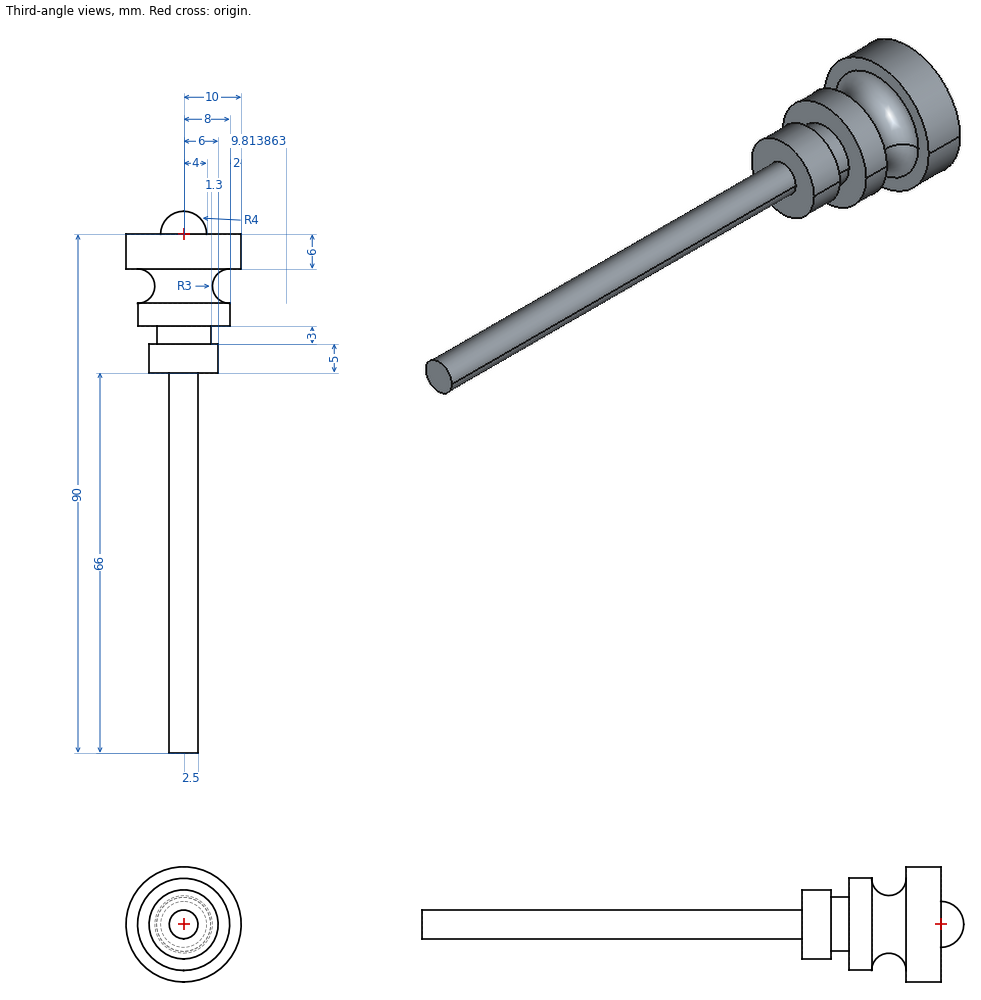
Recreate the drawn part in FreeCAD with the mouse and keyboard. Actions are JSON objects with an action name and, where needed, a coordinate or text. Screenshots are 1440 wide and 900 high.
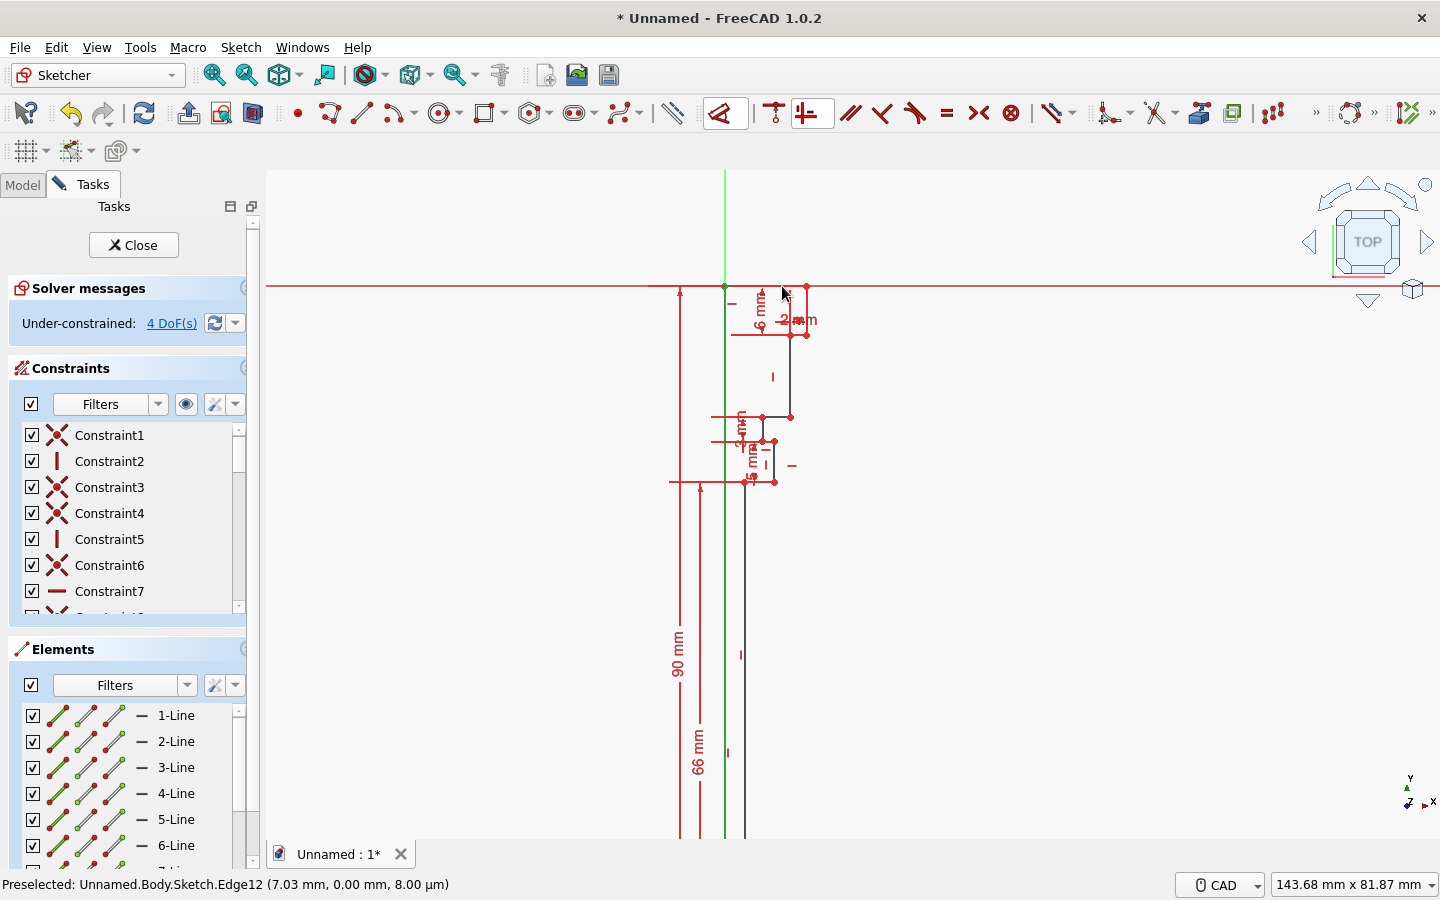
{"action": "key", "text": "l"}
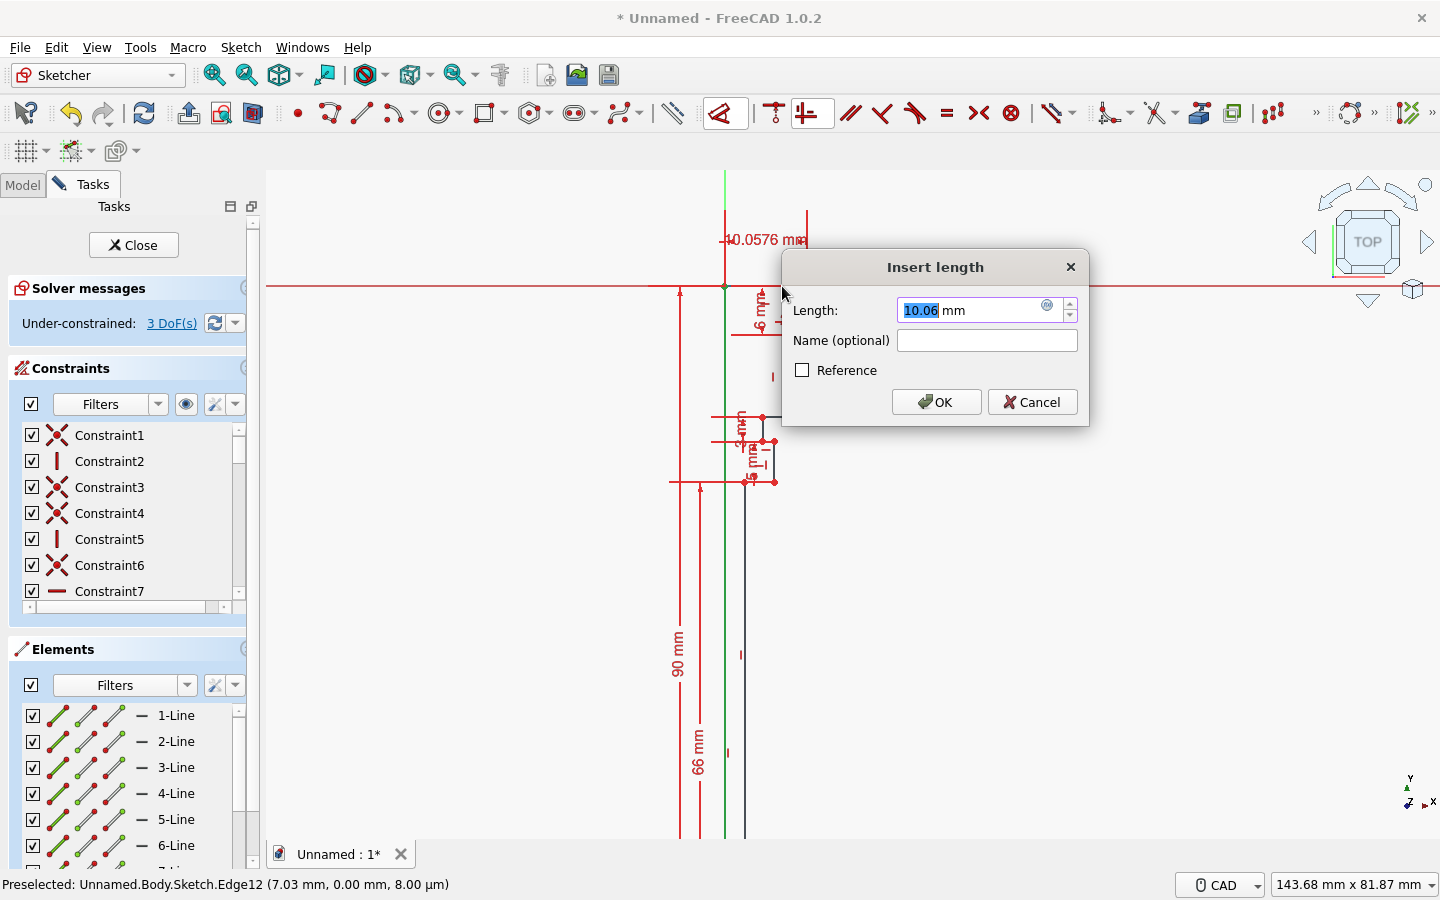
{"action": "type", "text": "10"}
{"action": "key", "text": "Return"}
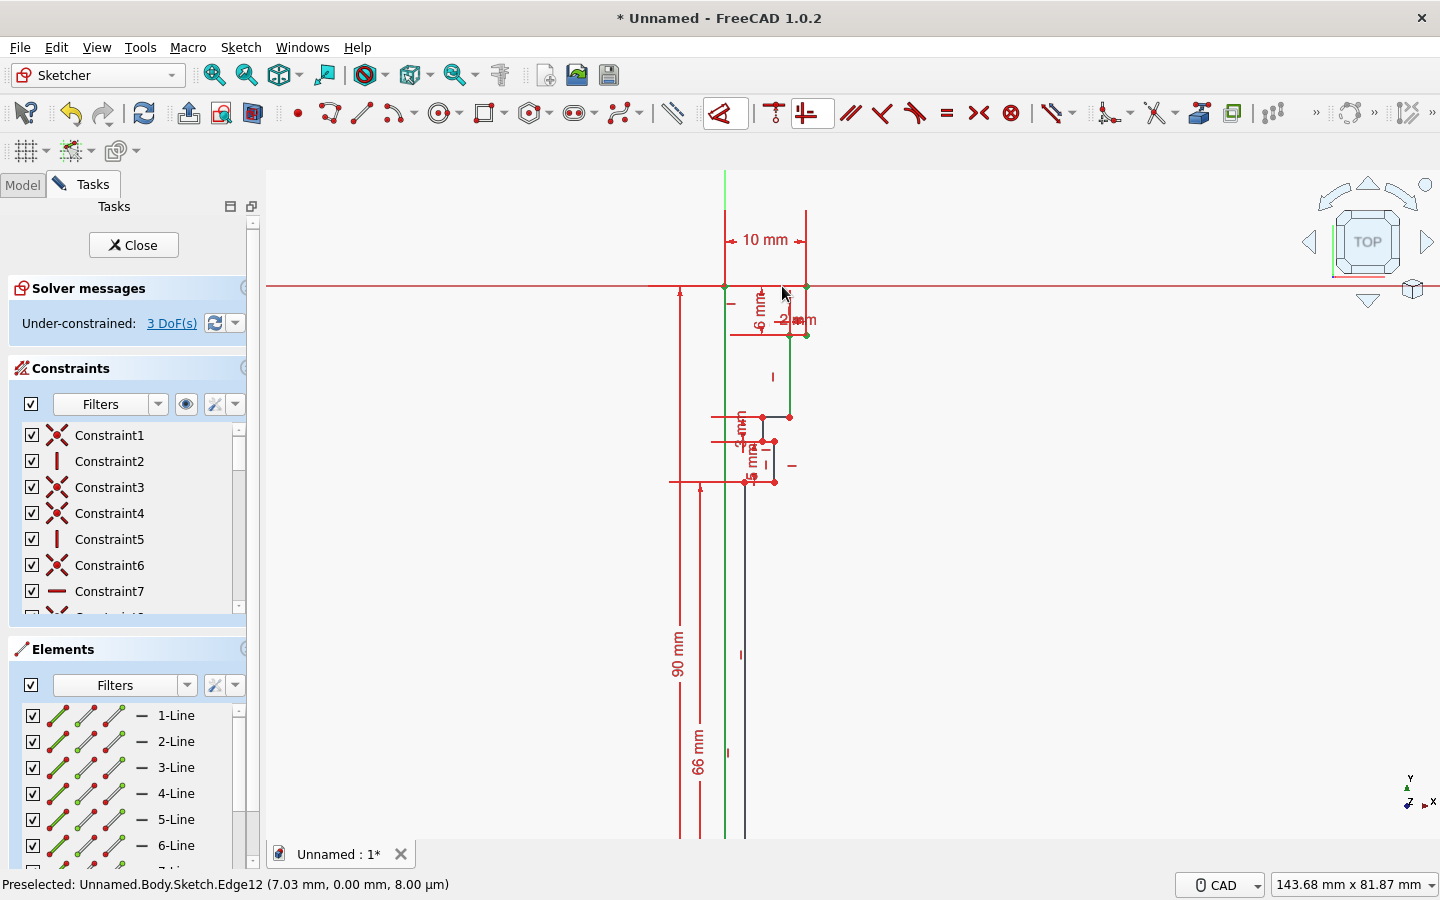
{"action": "left_click", "coordinate": [774, 482]}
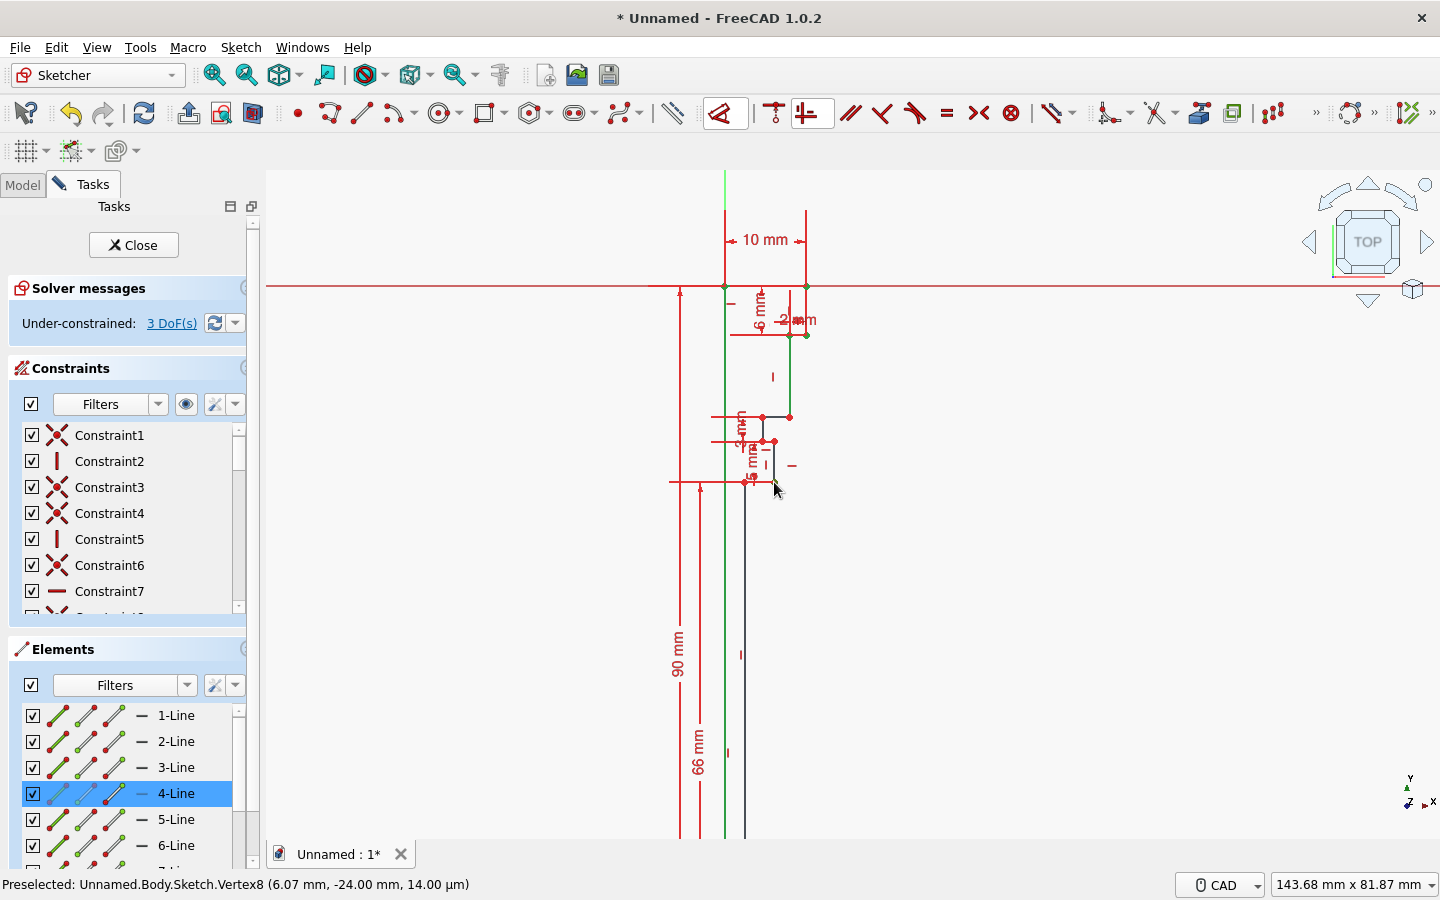
{"action": "key", "text": "l"}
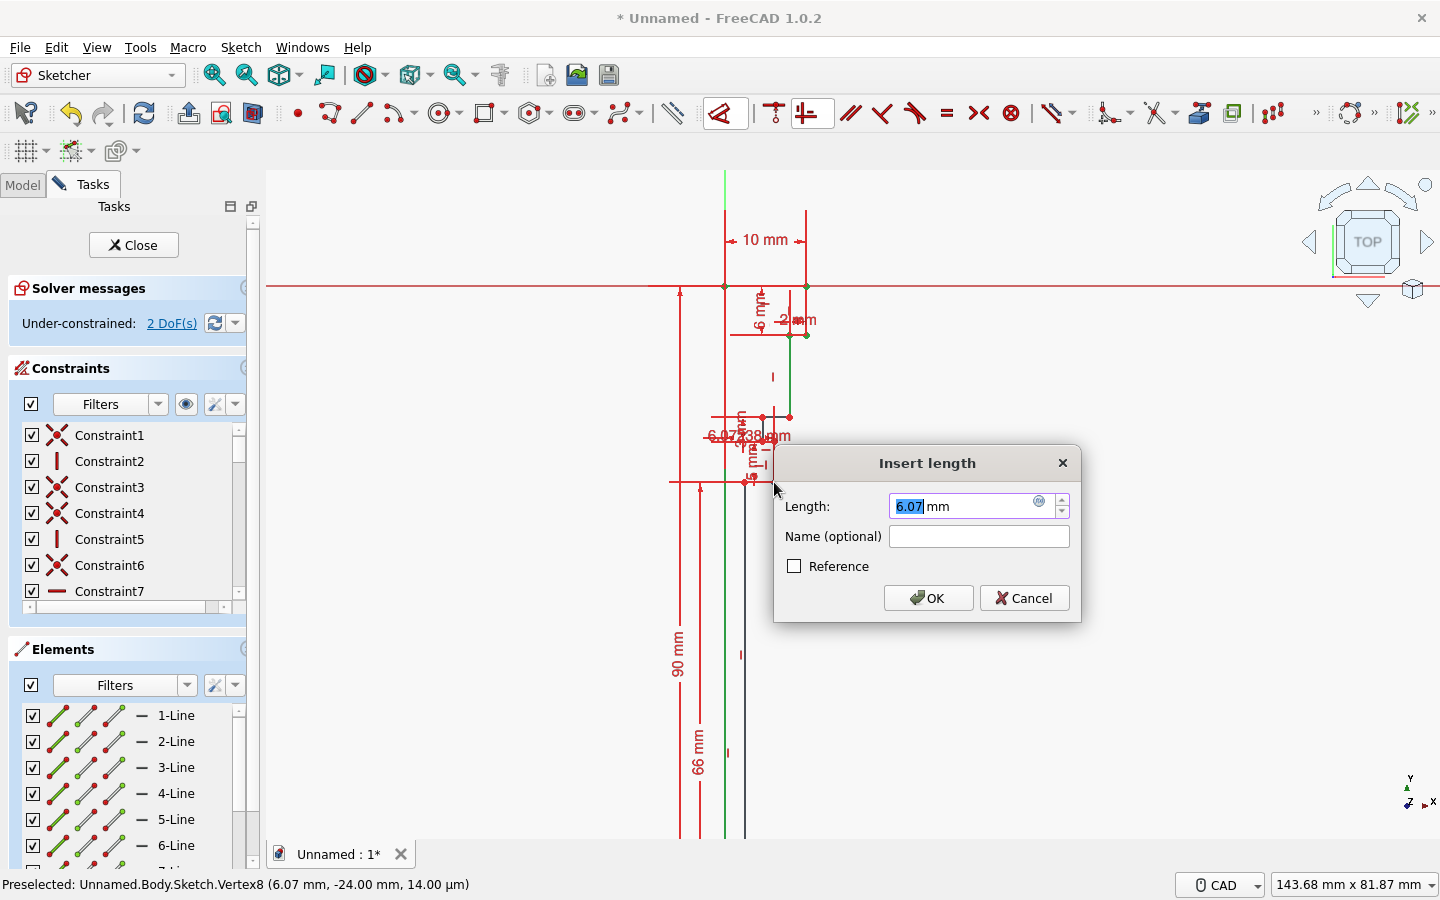
{"action": "type", "text": "6"}
{"action": "key", "text": "Return"}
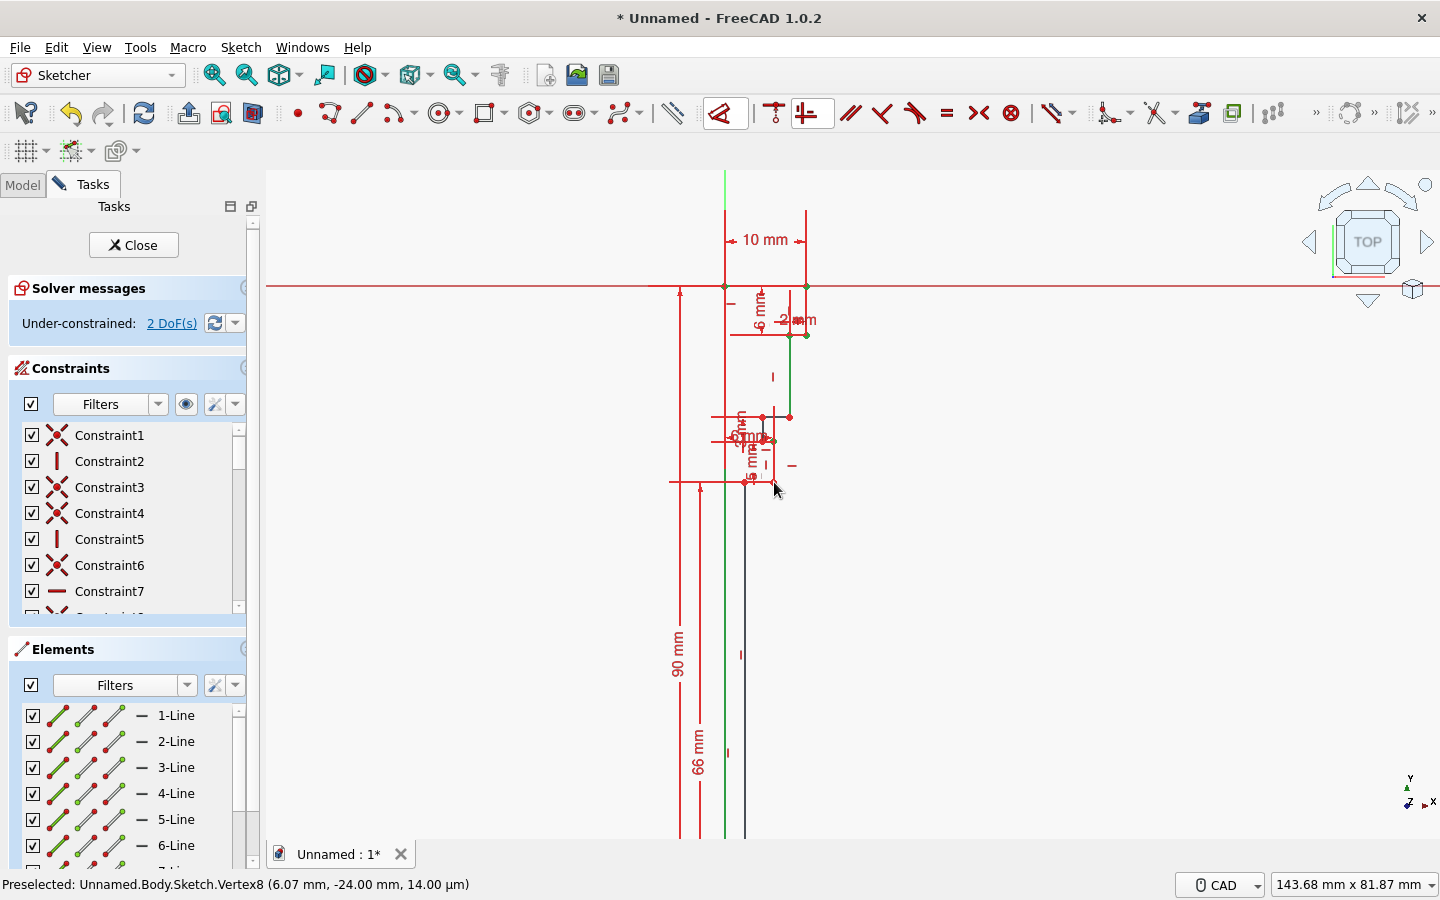
{"action": "scroll", "coordinate": [808, 323], "scroll_direction": "down", "scroll_amount": 3}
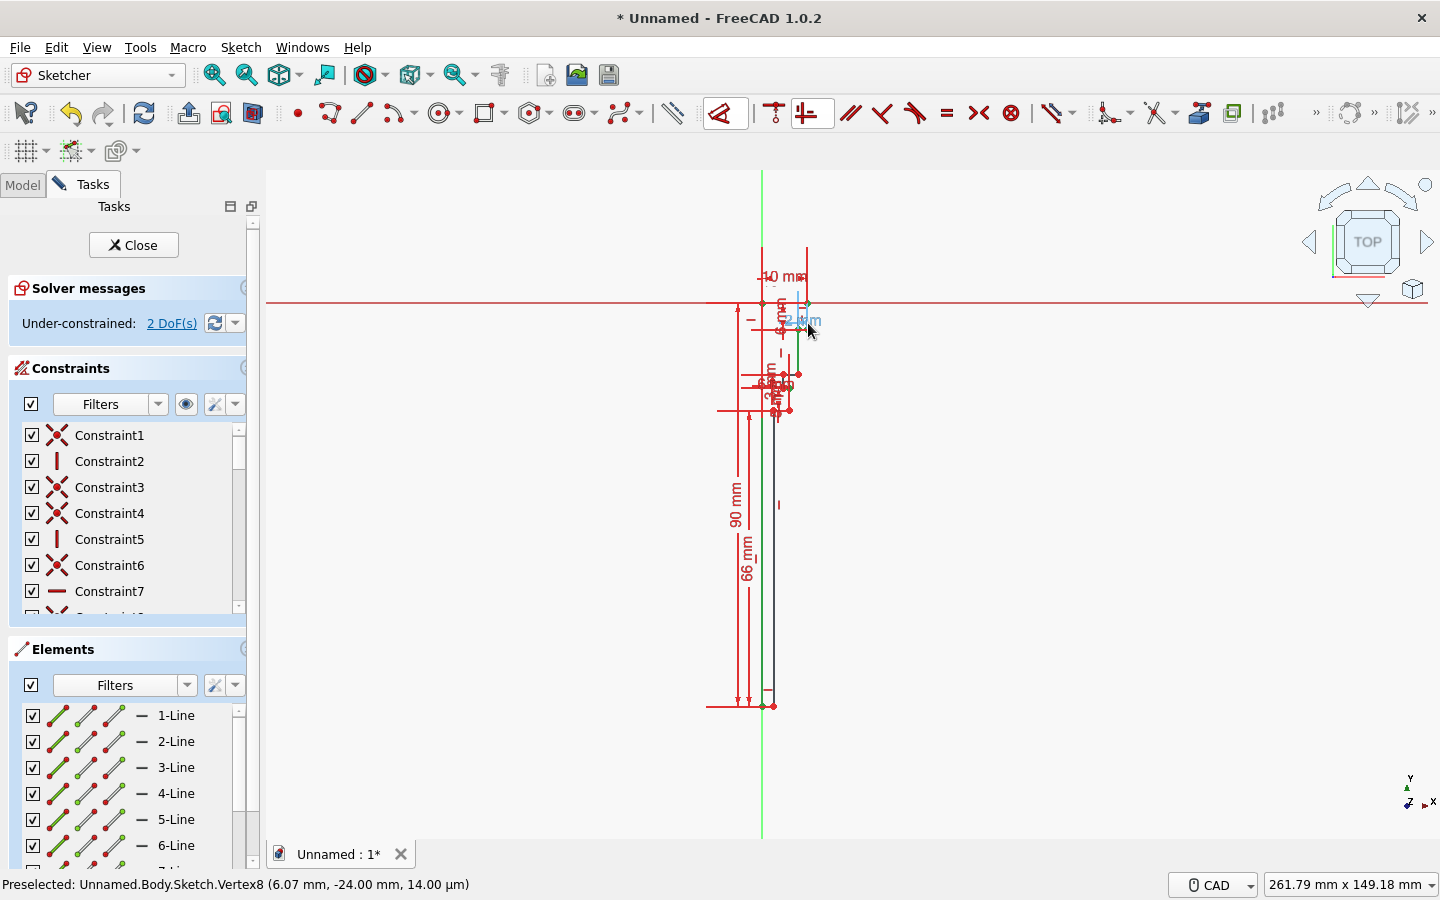
{"action": "scroll", "coordinate": [768, 707], "scroll_direction": "up", "scroll_amount": 7}